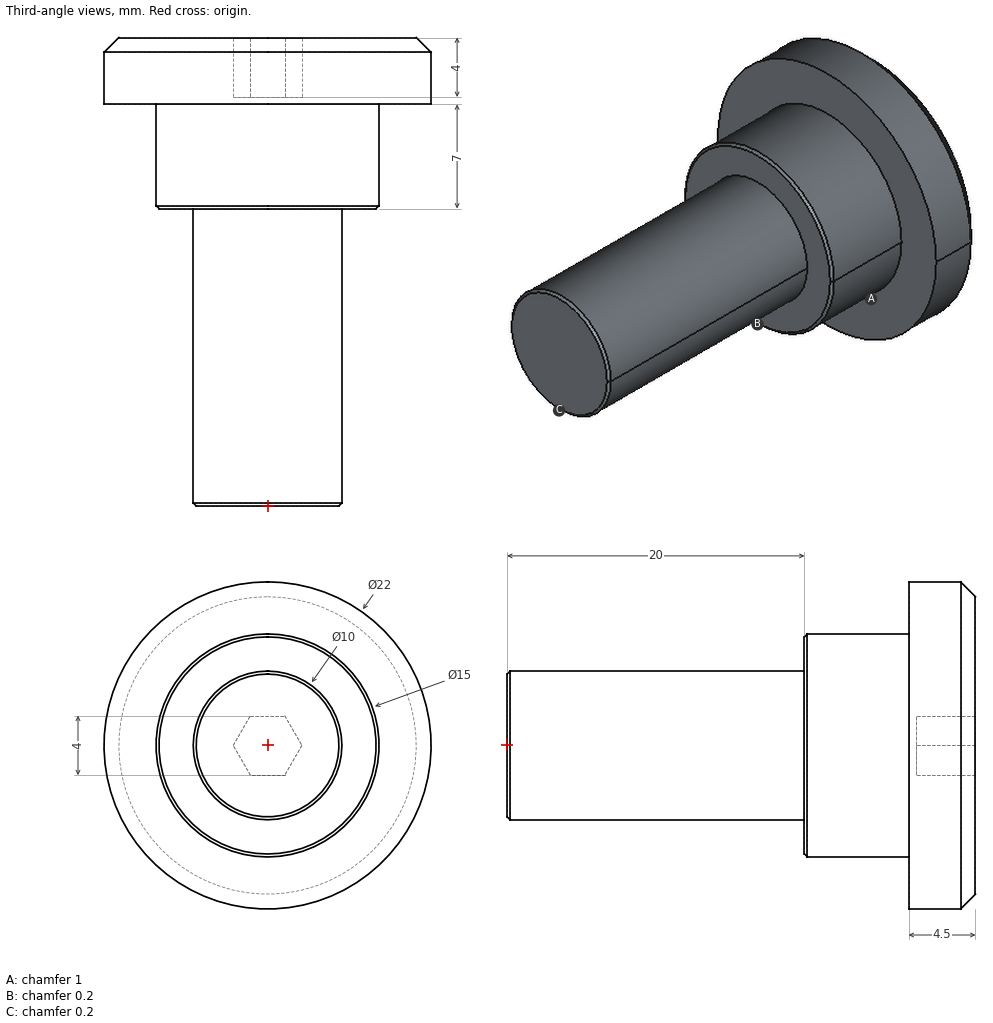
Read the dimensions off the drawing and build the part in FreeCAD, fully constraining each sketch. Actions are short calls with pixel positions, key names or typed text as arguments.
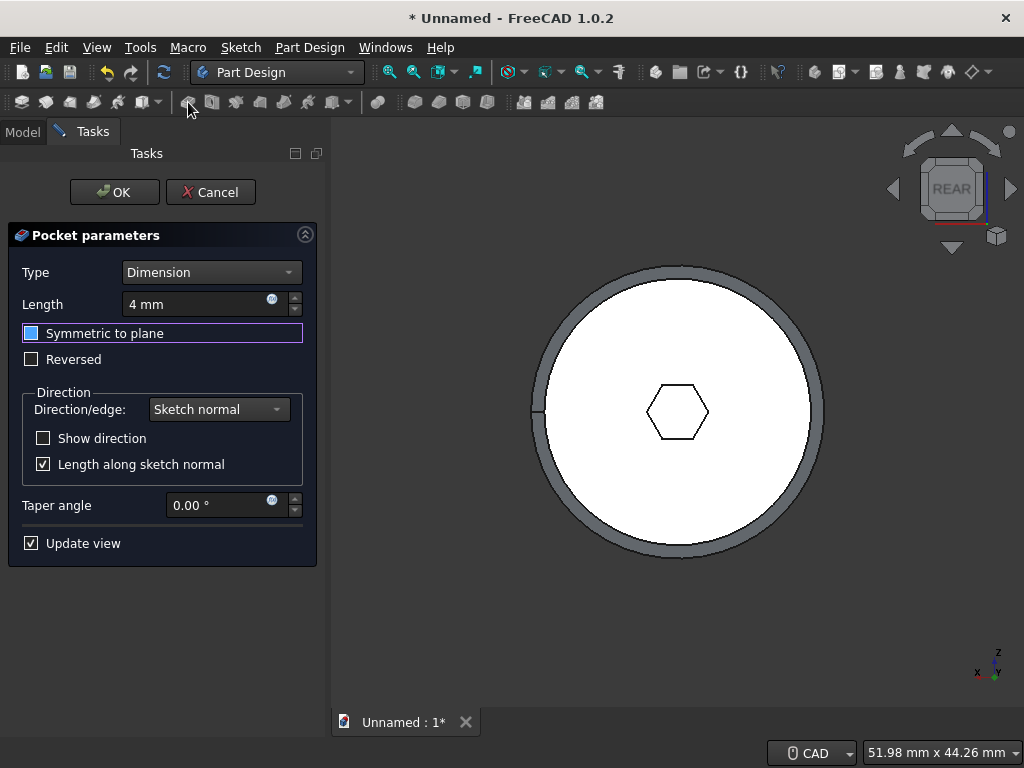
click(115, 192)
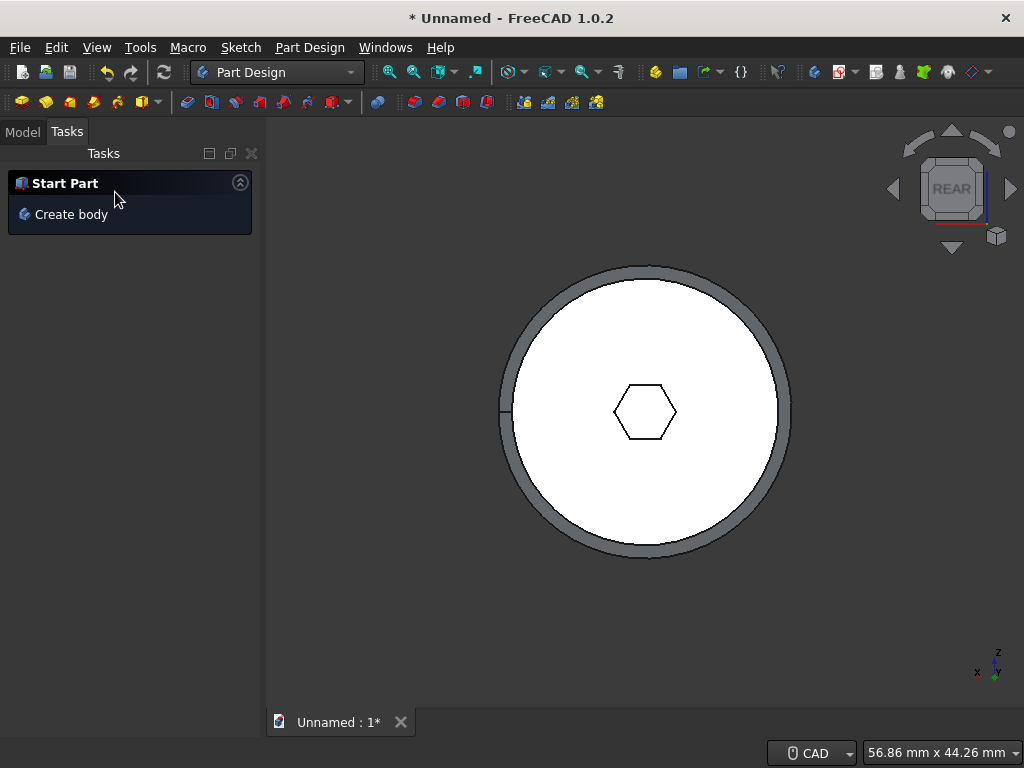
key(0)